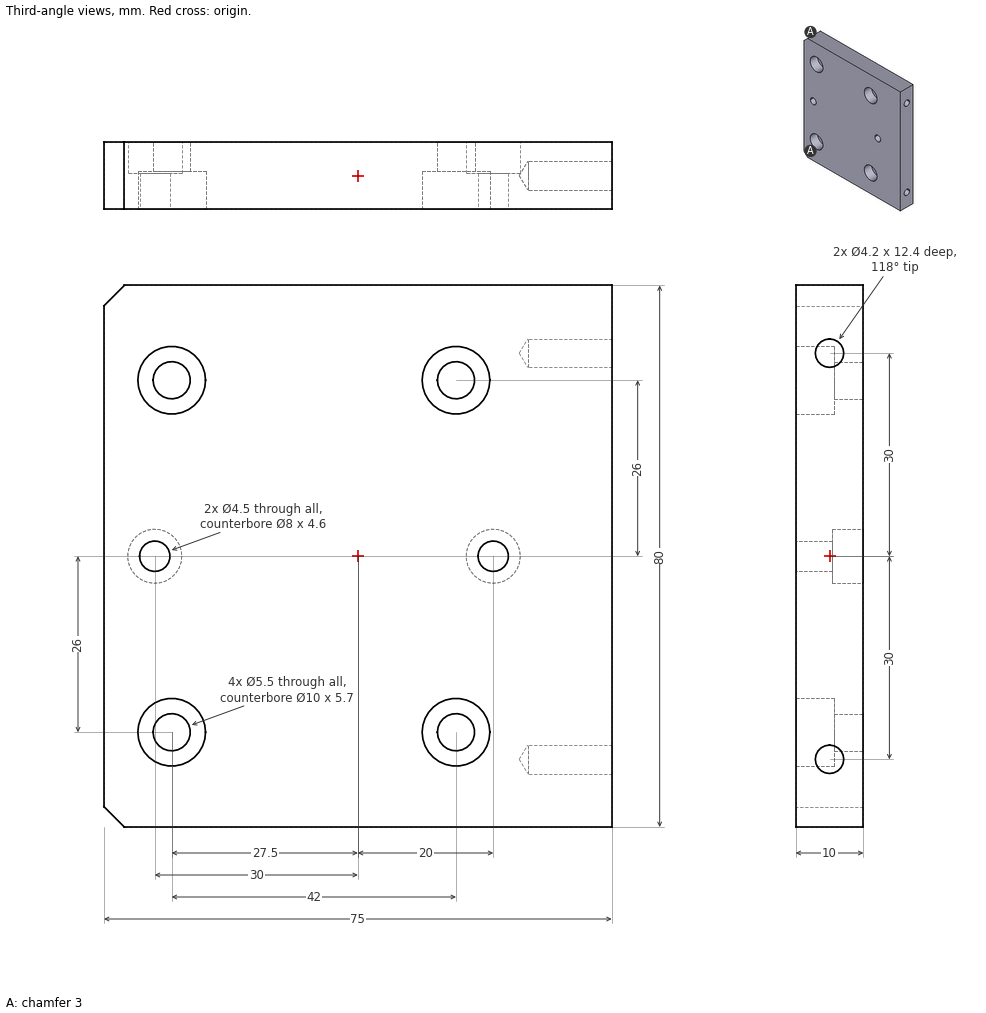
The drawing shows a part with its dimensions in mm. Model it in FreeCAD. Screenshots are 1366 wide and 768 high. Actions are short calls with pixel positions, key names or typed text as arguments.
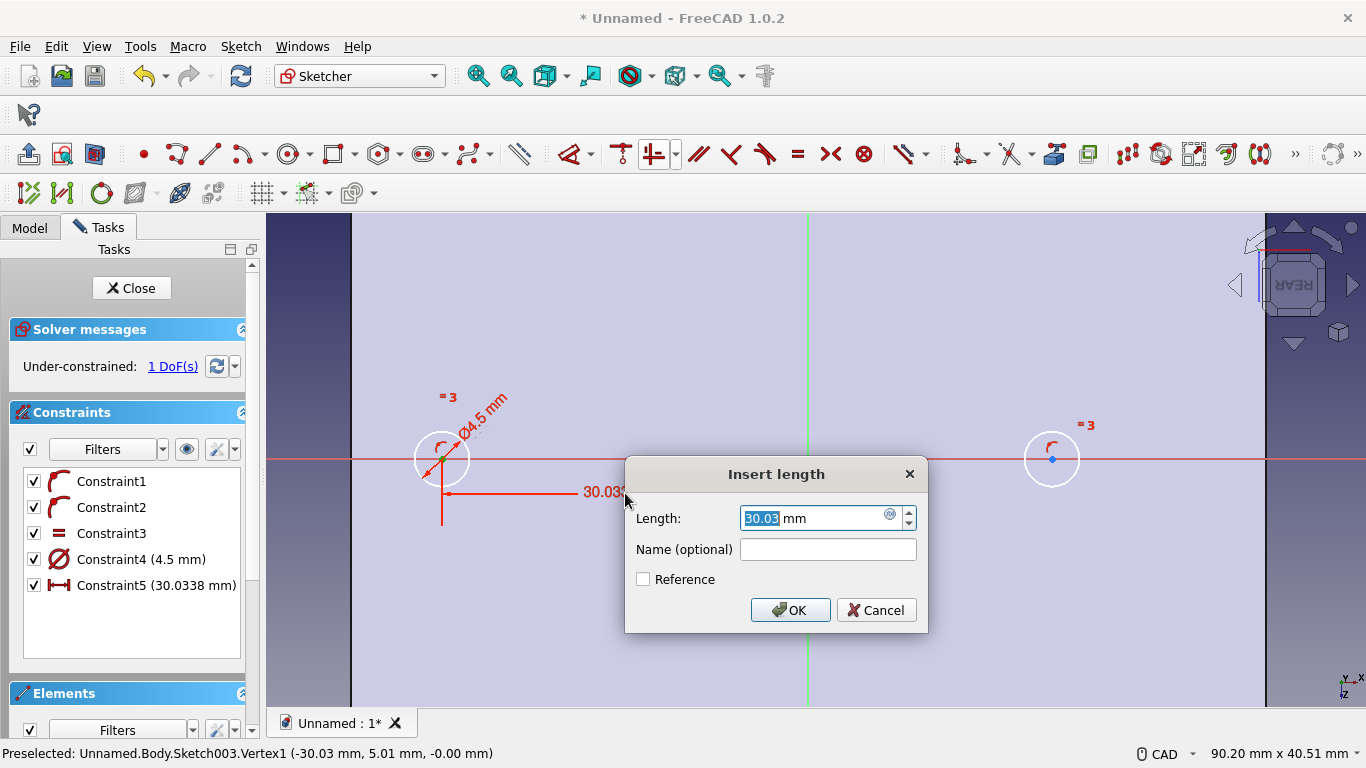
text(30)
key(Return)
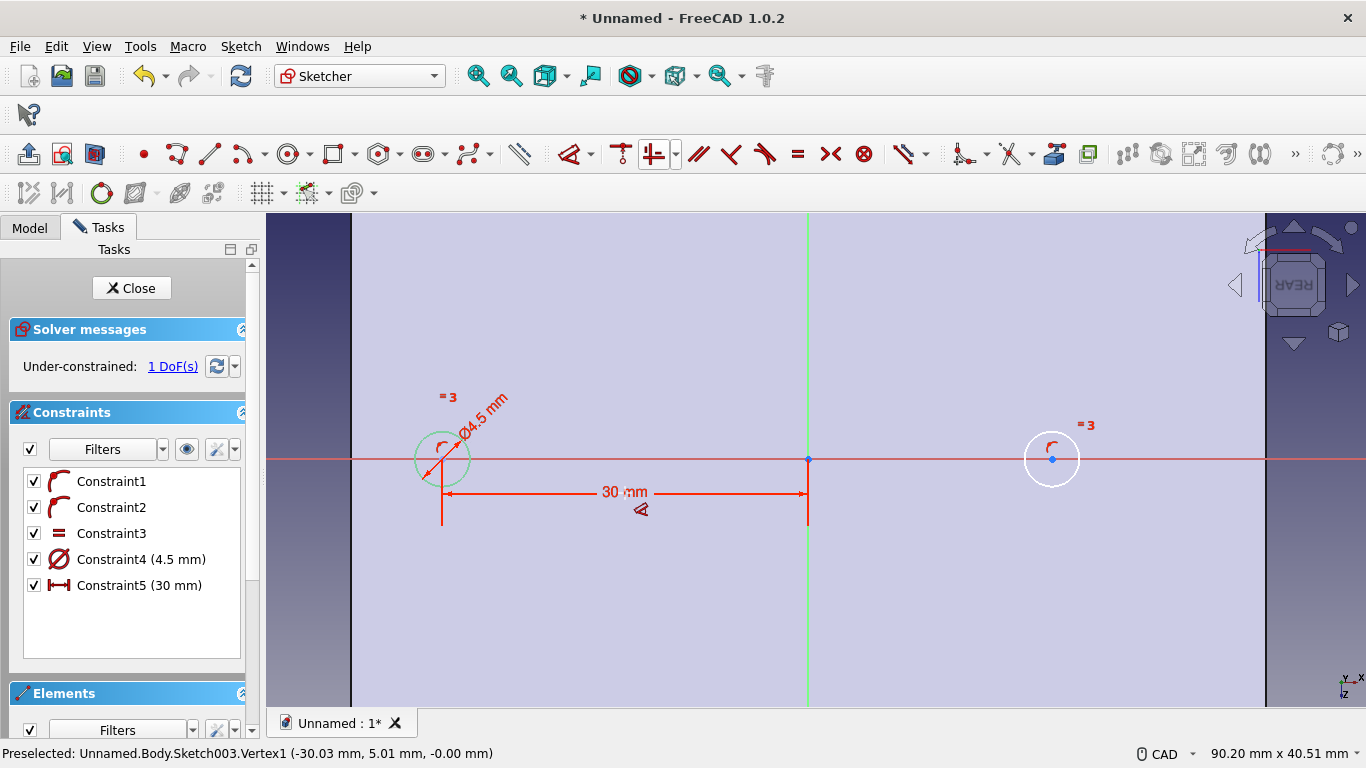
click(1052, 459)
click(930, 493)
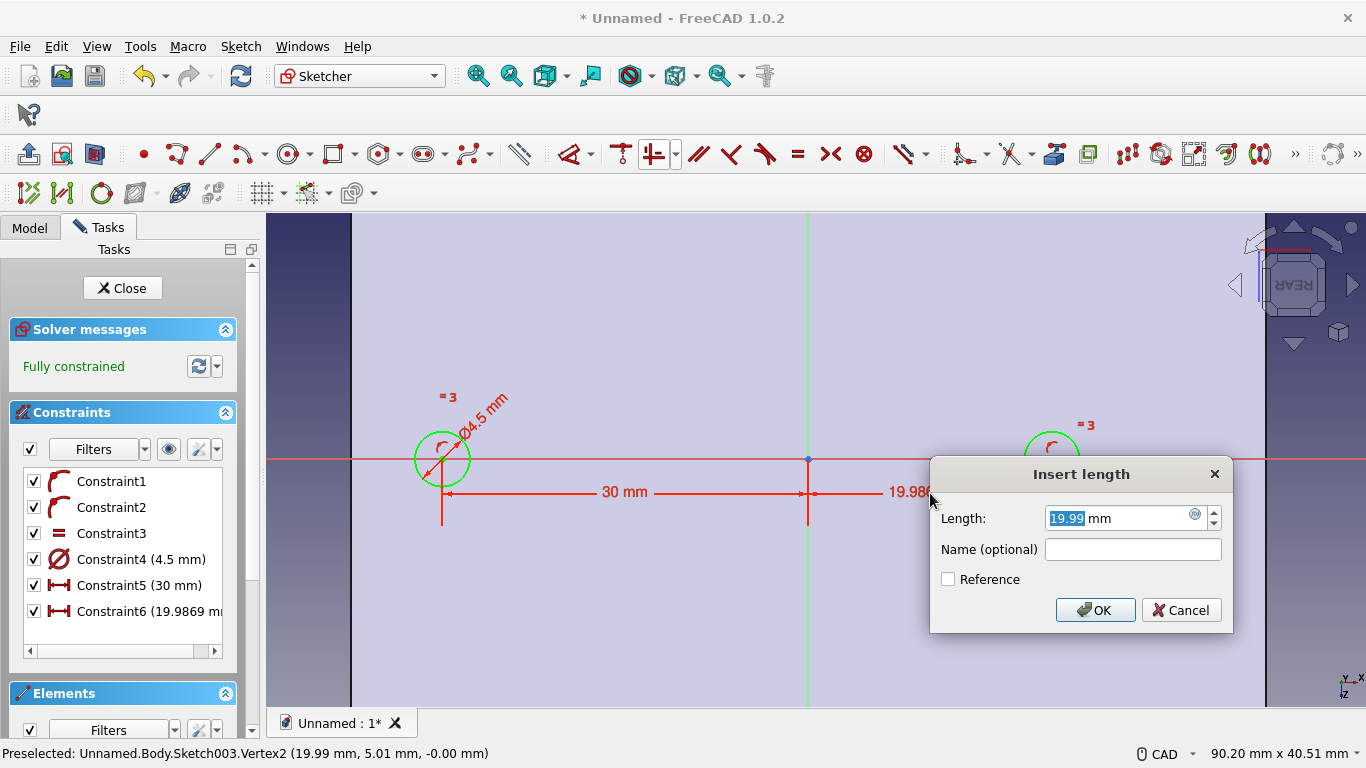
text(20)
key(Return)
key(Escape)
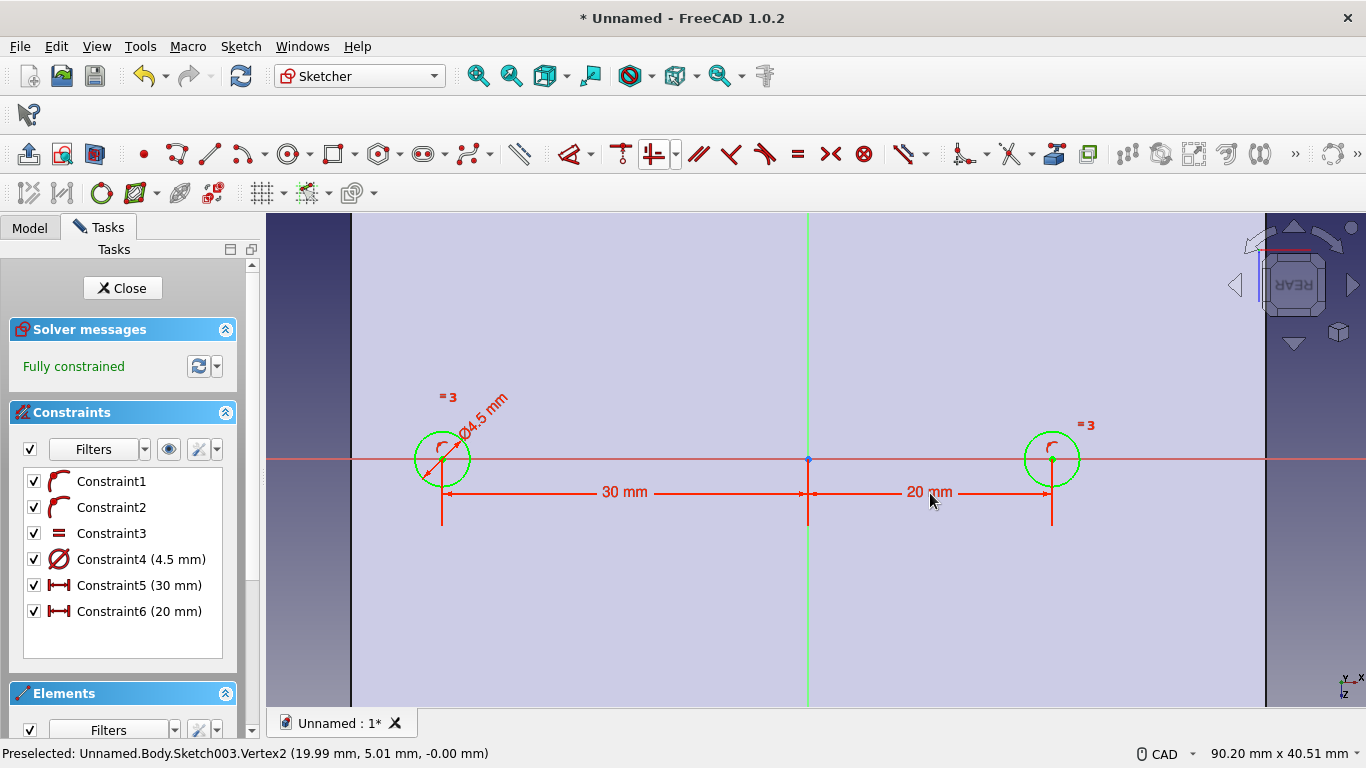
click(123, 288)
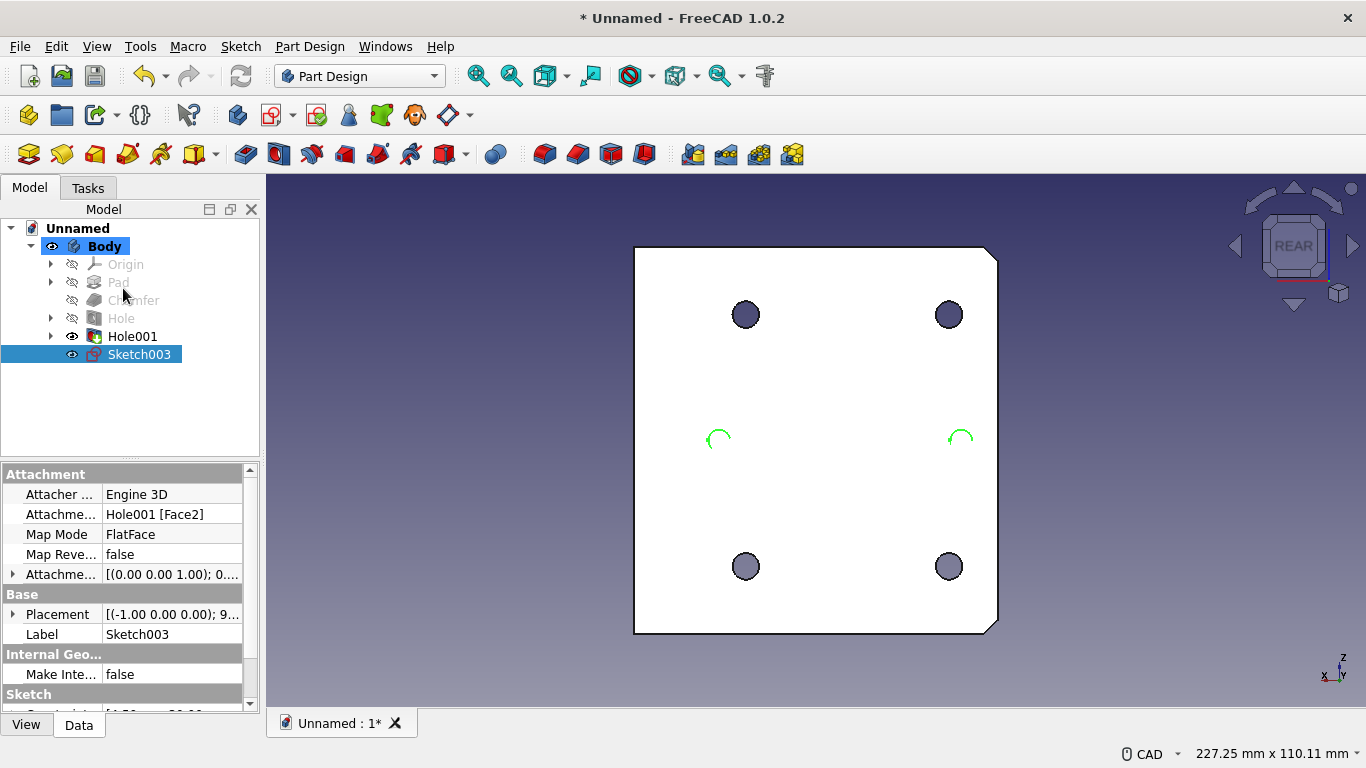
click(279, 154)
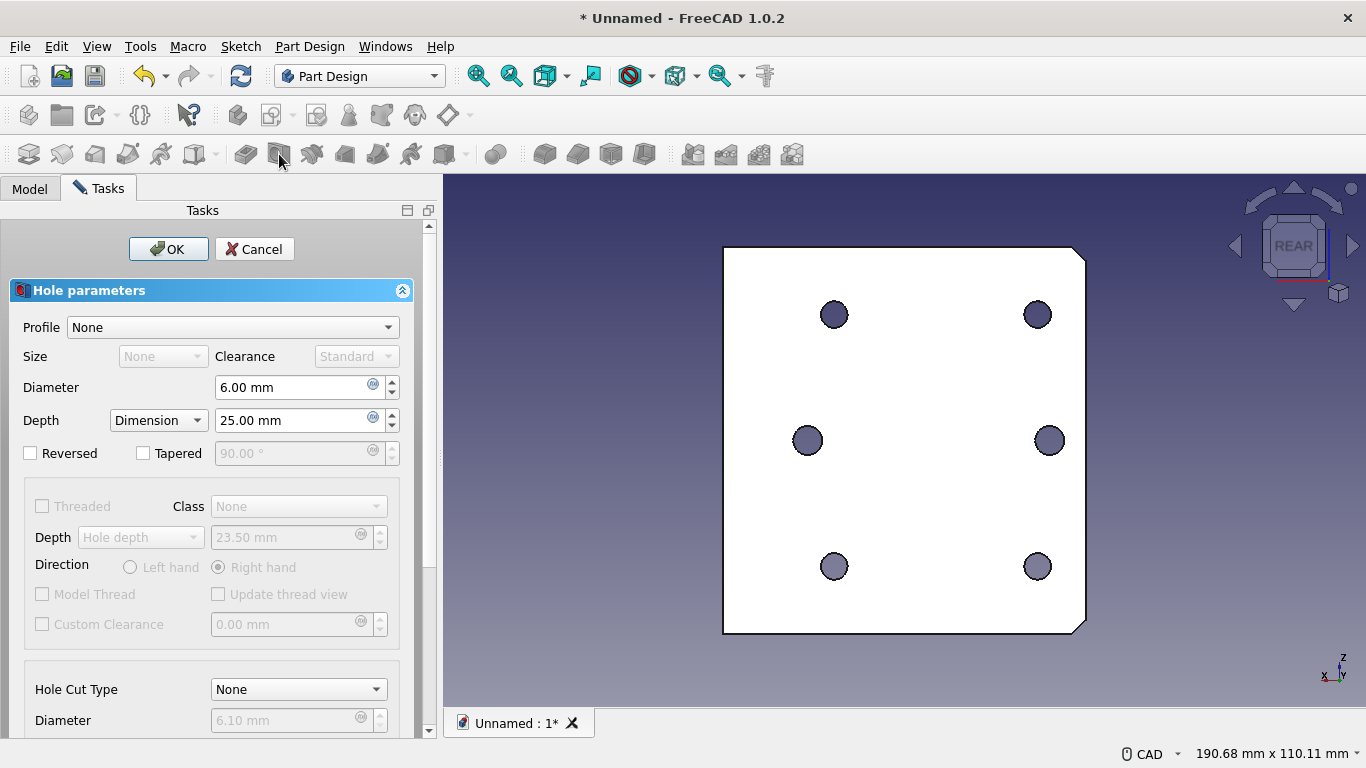
triple_click(300, 388)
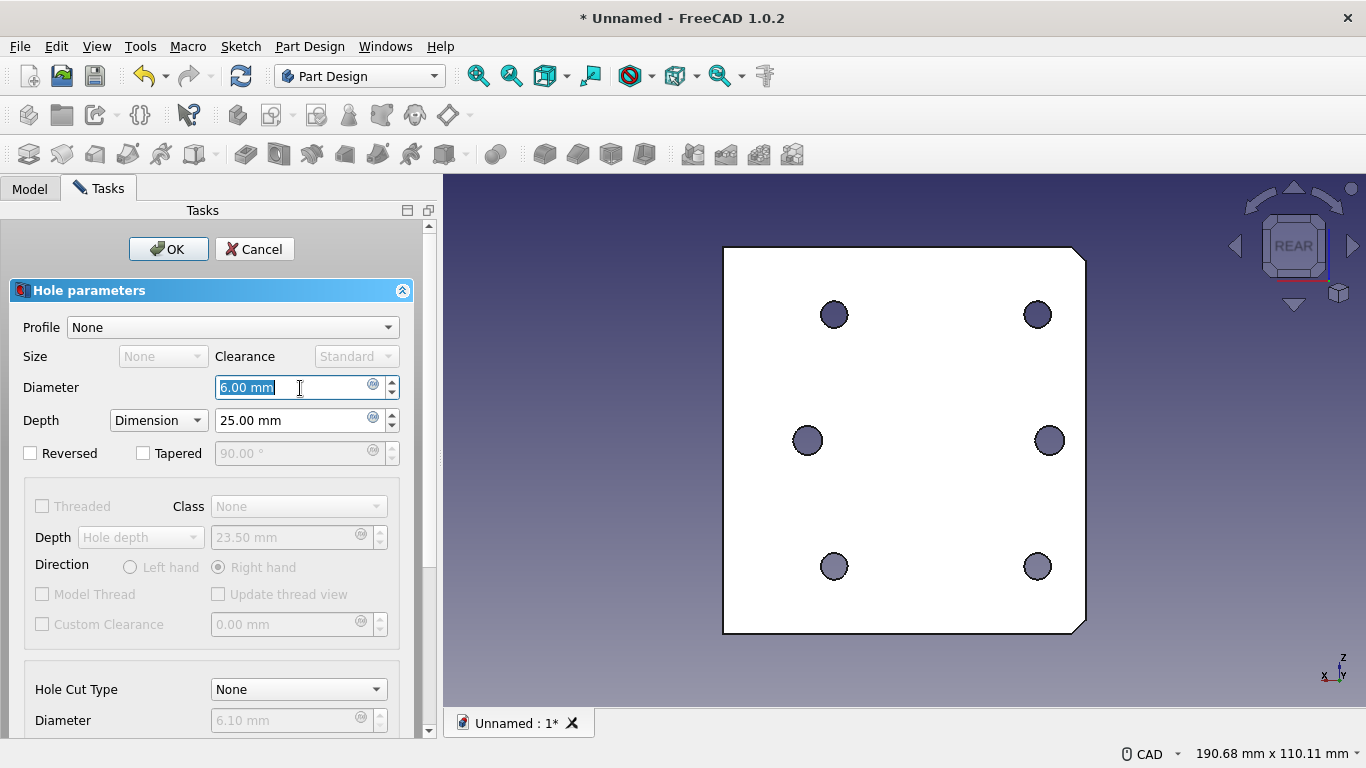
text(4.5)
key(Tab)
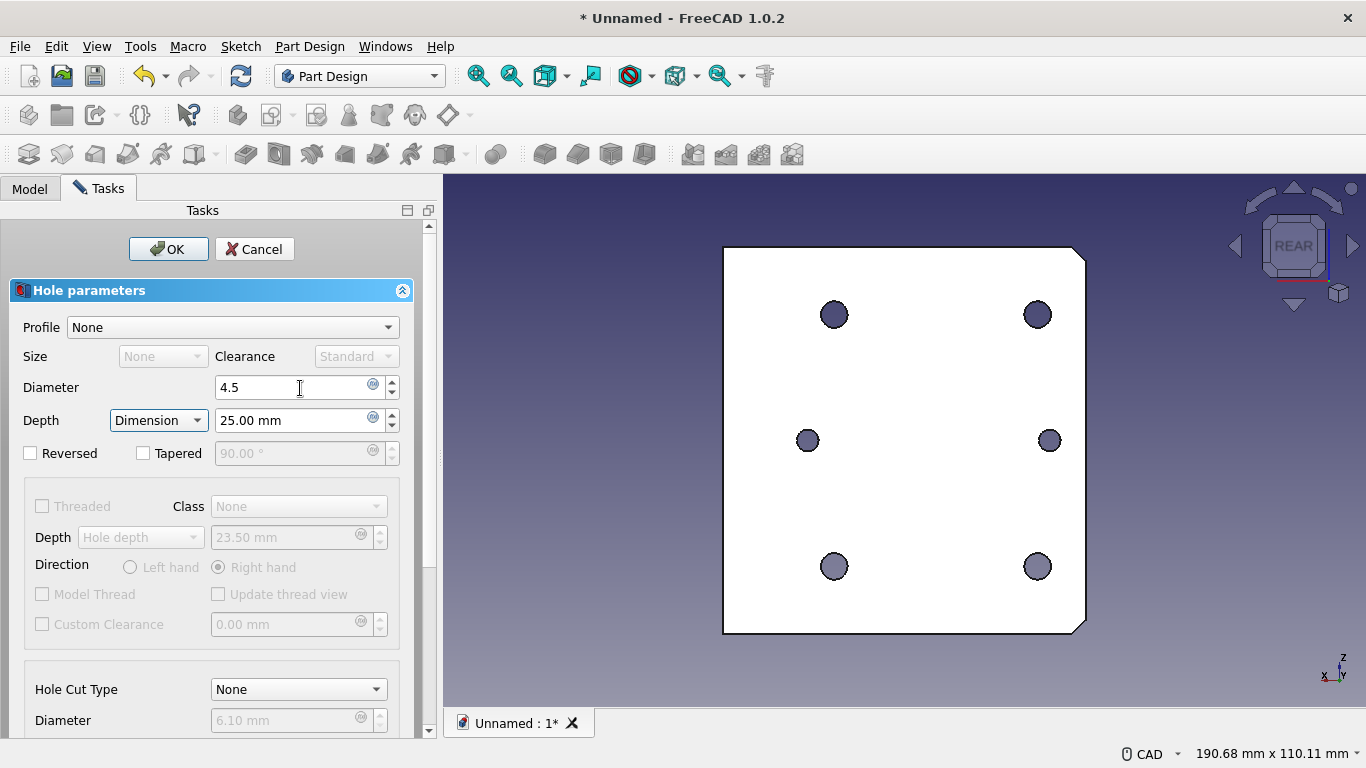
click(160, 420)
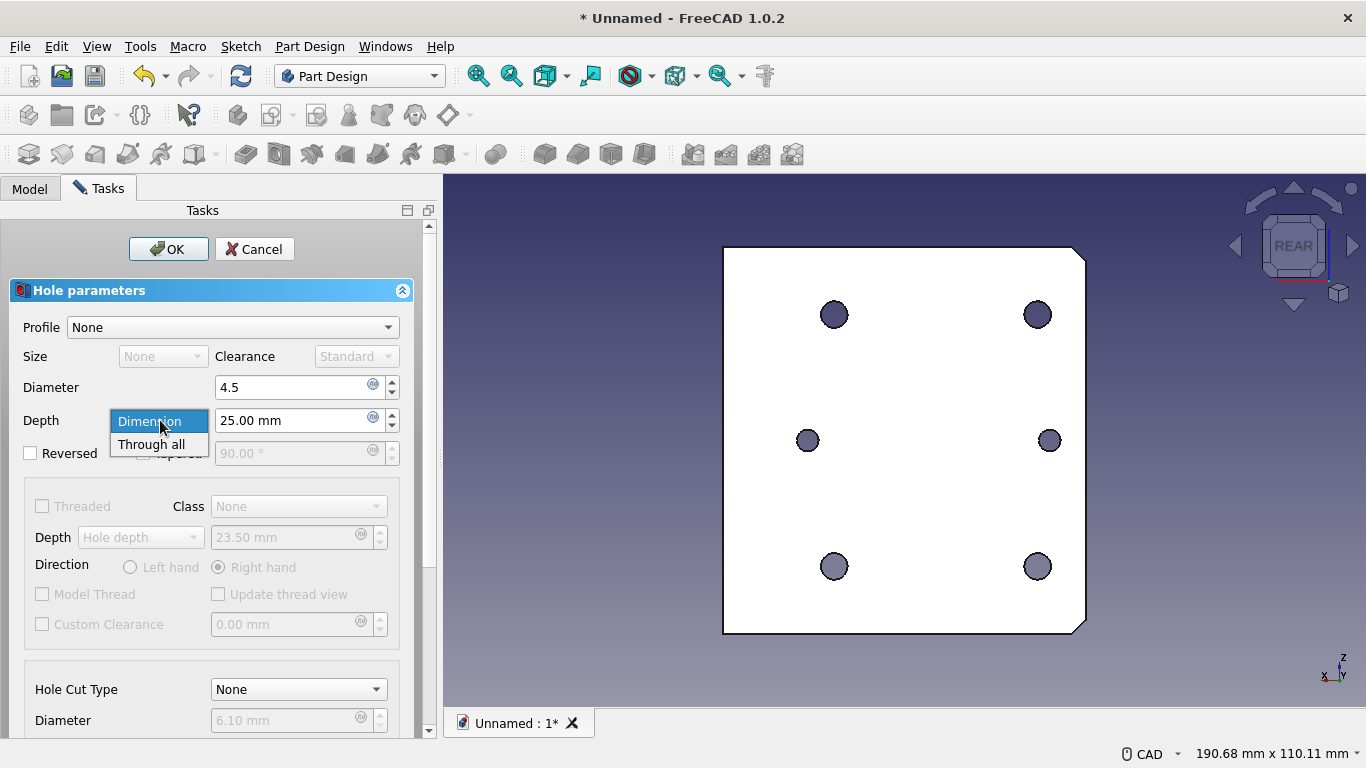
click(158, 444)